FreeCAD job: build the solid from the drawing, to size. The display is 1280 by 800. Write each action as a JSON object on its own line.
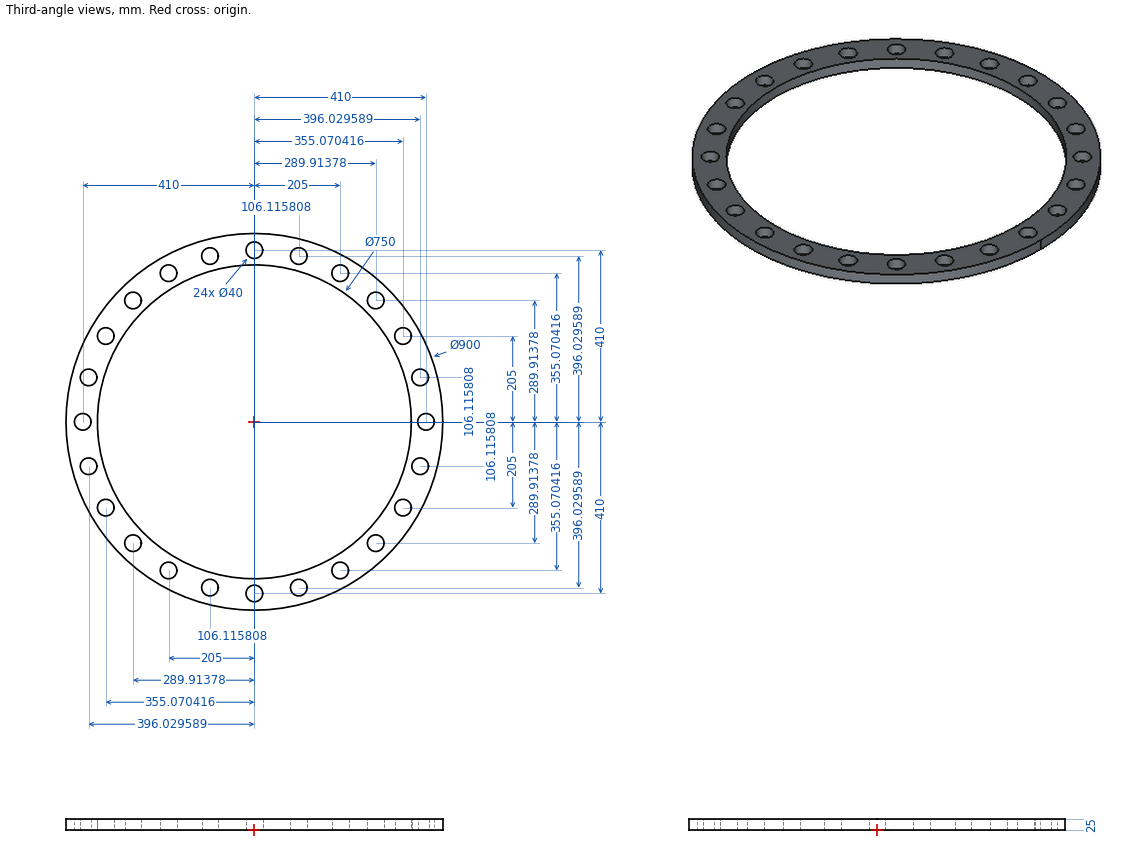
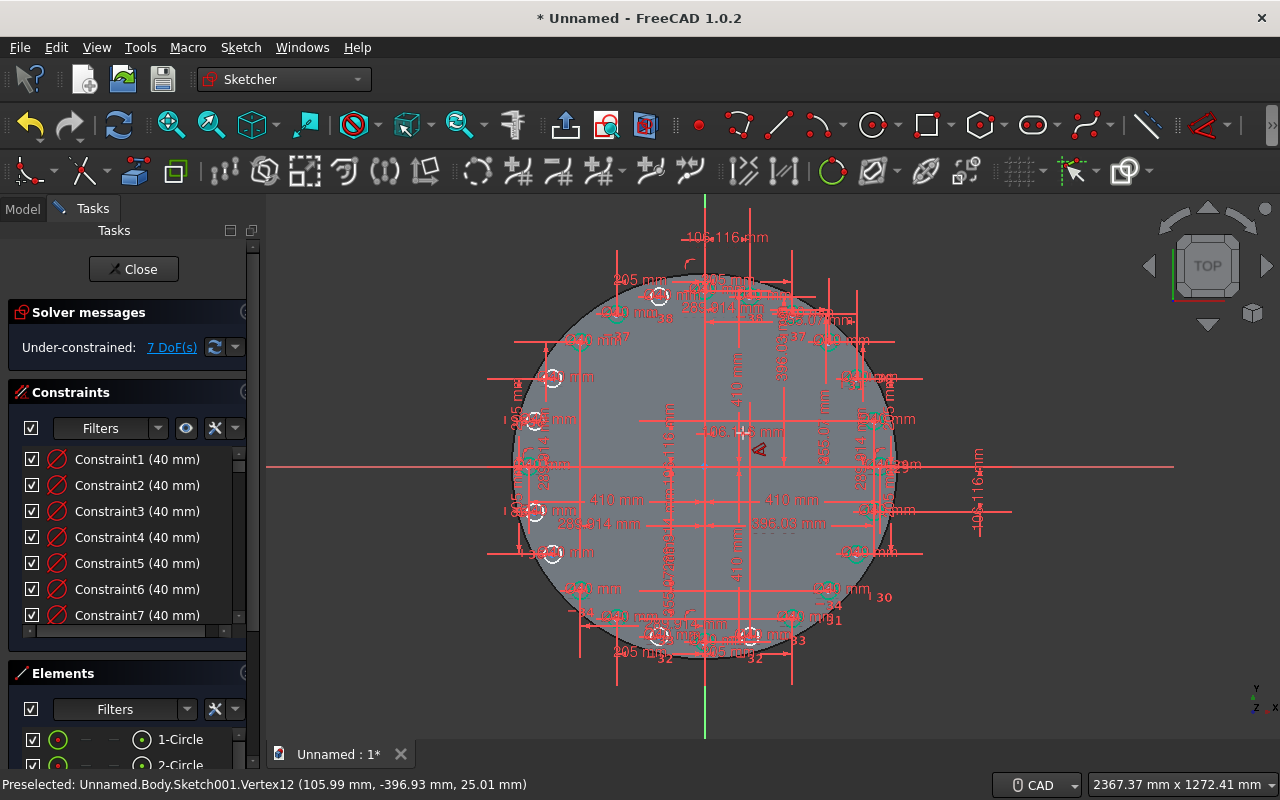
{"action": "left_click", "coordinate": [750, 637]}
{"action": "left_click", "coordinate": [784, 591]}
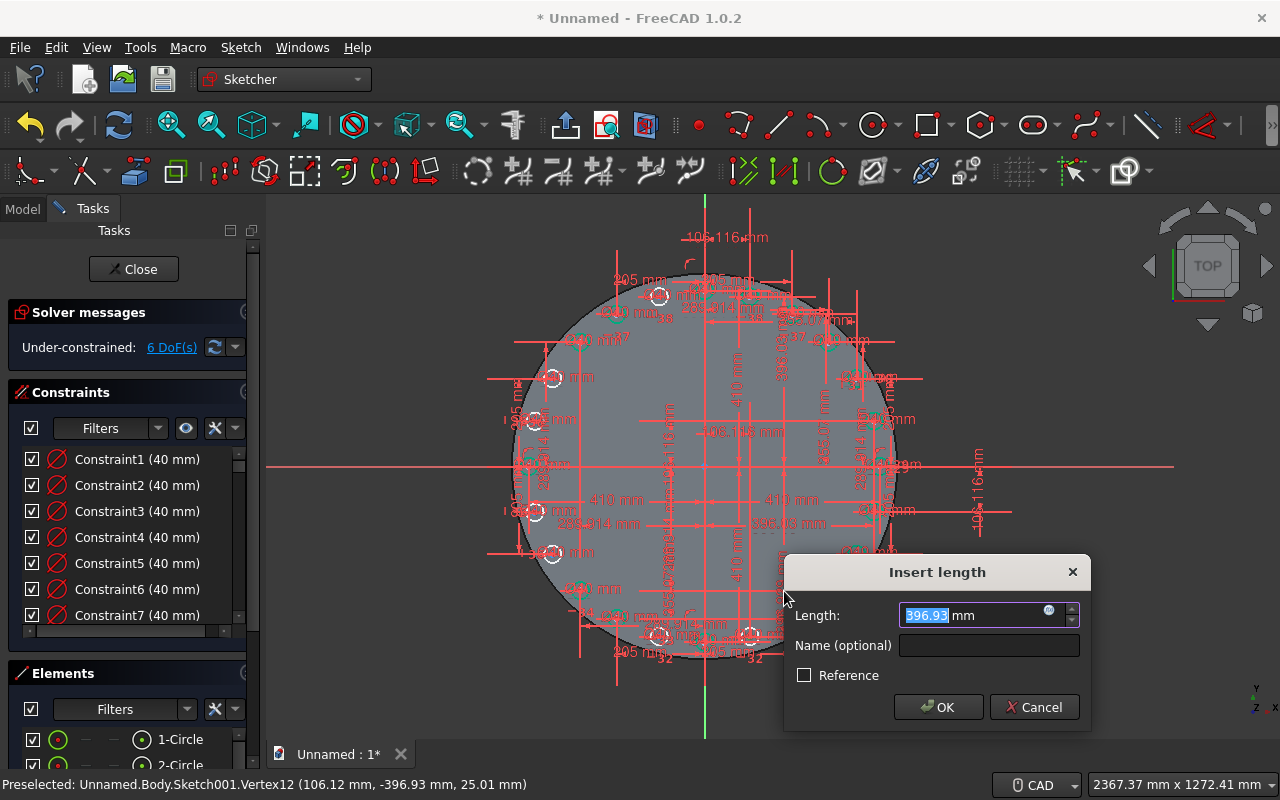
{"action": "type", "text": "396.029589"}
{"action": "key", "text": "Return"}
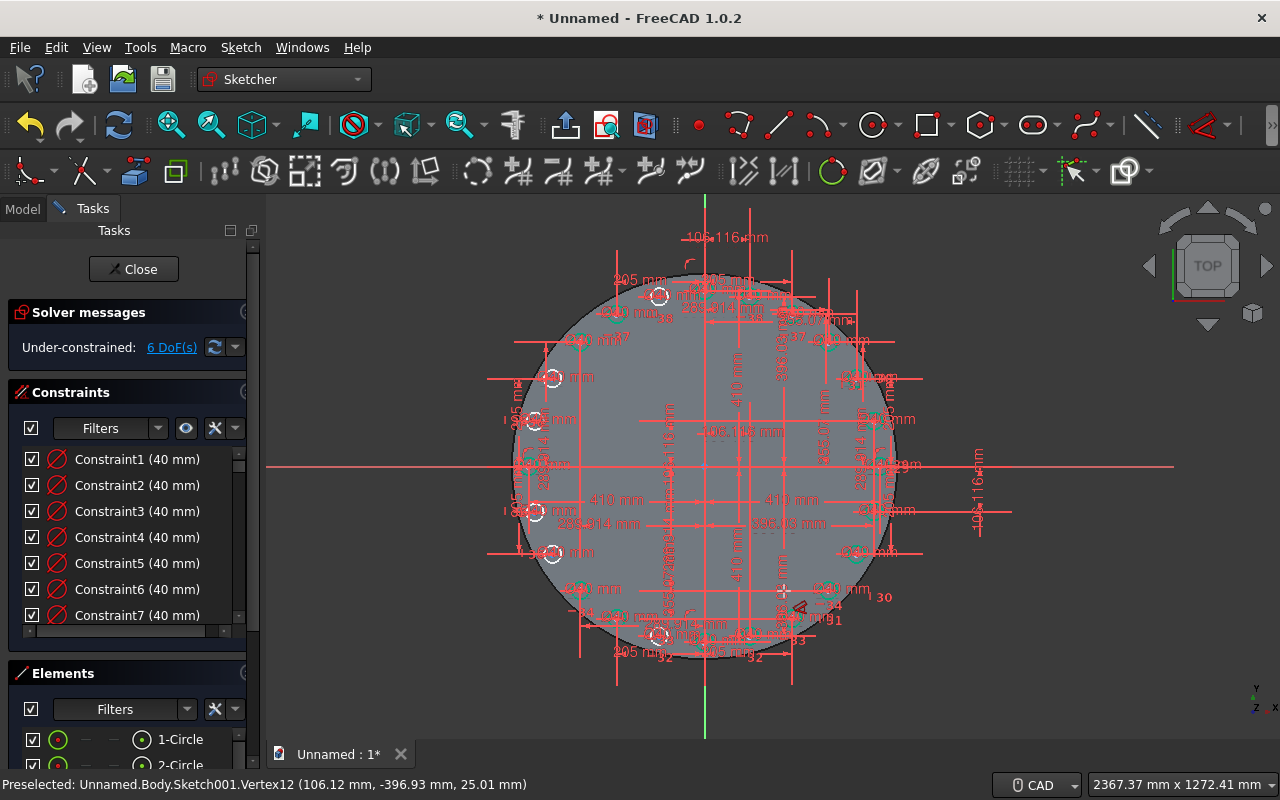
{"action": "left_click", "coordinate": [659, 636]}
{"action": "left_click", "coordinate": [682, 694]}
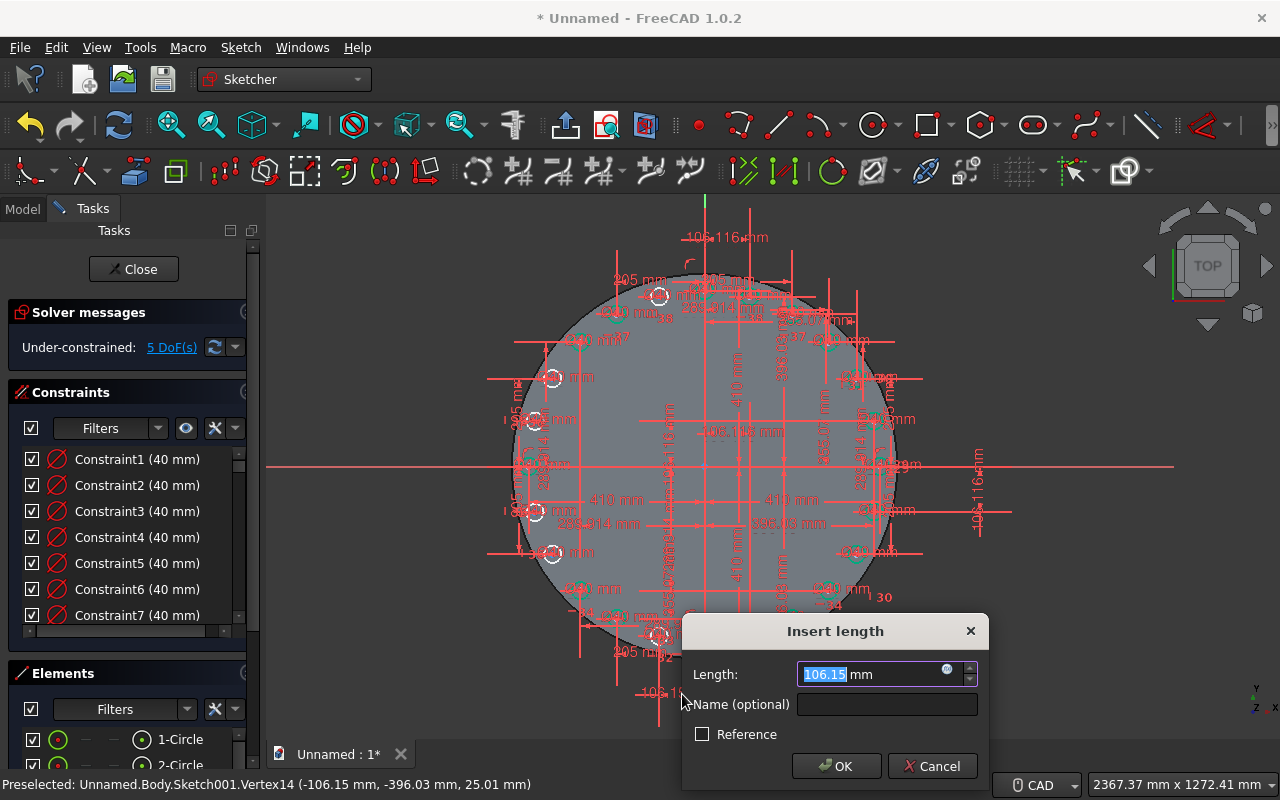
{"action": "type", "text": "106.115808"}
{"action": "key", "text": "Return"}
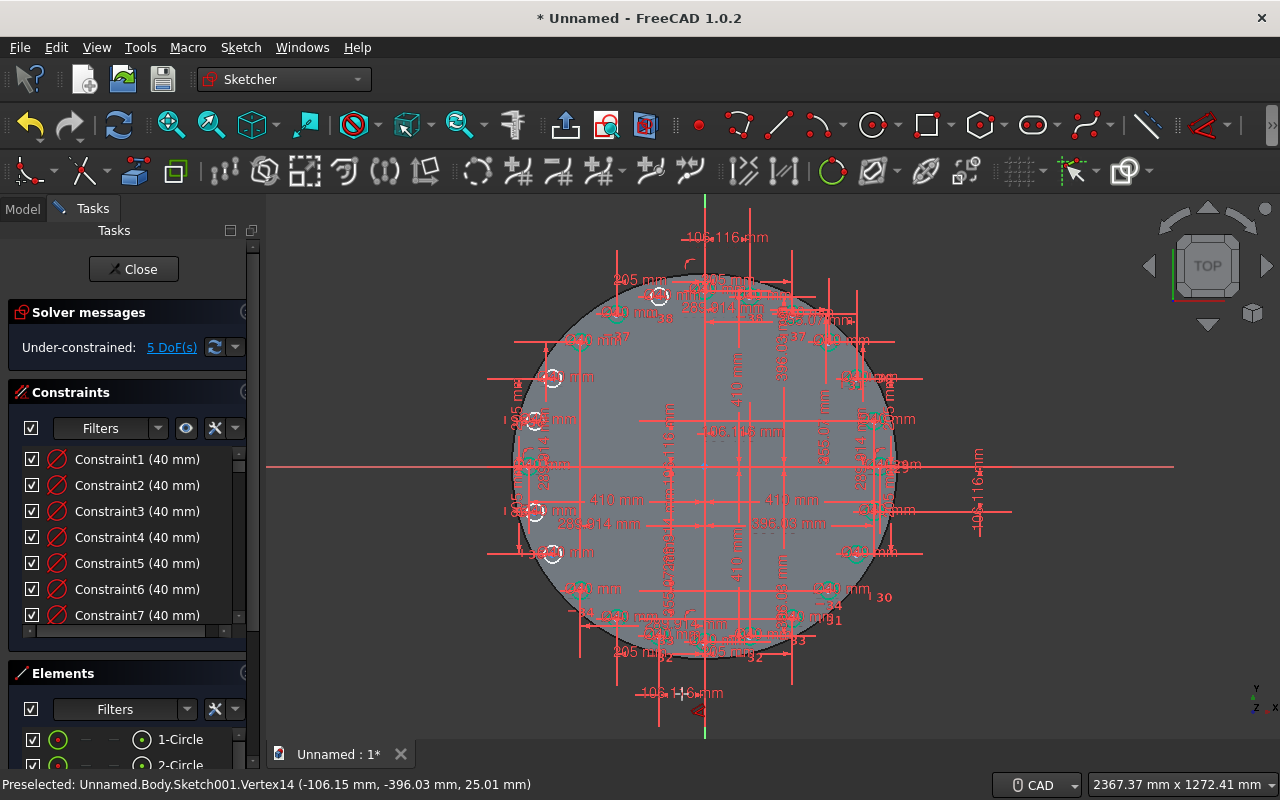
{"action": "left_click", "coordinate": [553, 554]}
{"action": "left_click", "coordinate": [594, 612]}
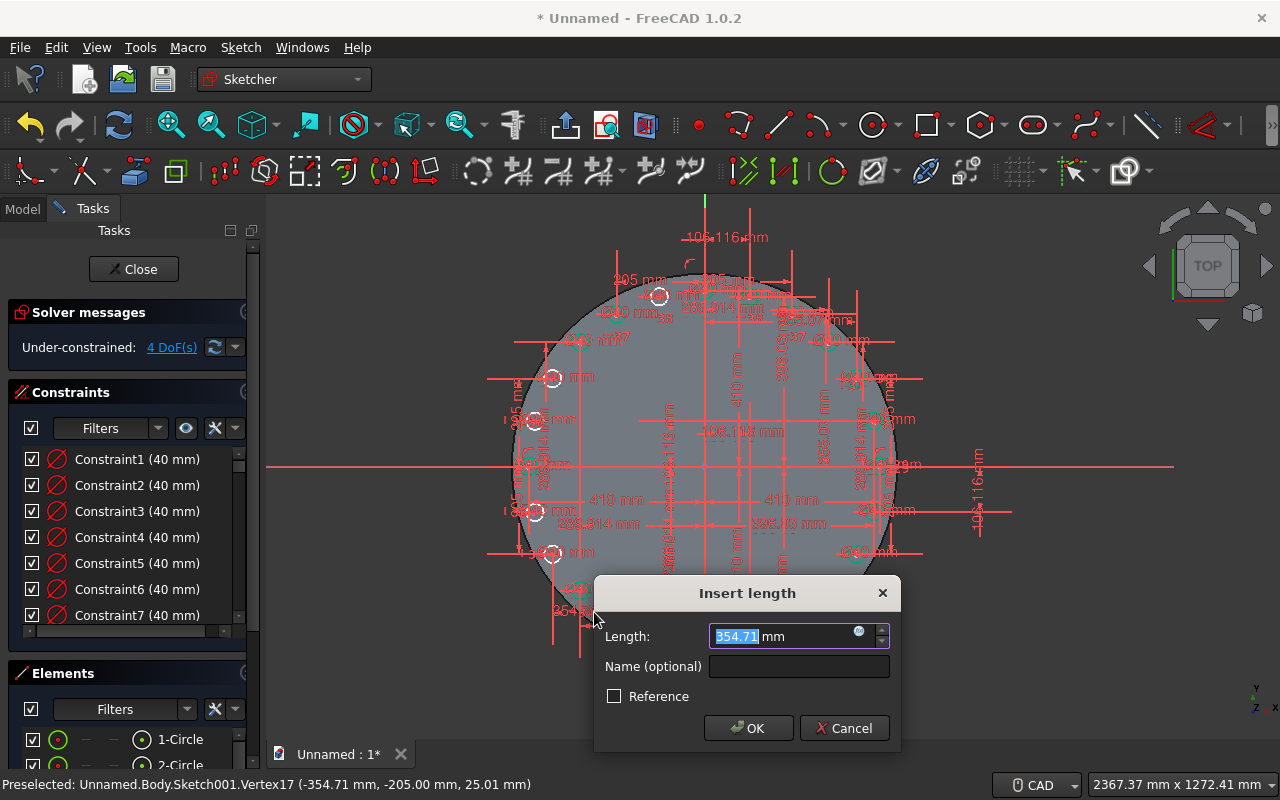
{"action": "type", "text": "355.070416"}
{"action": "key", "text": "Return"}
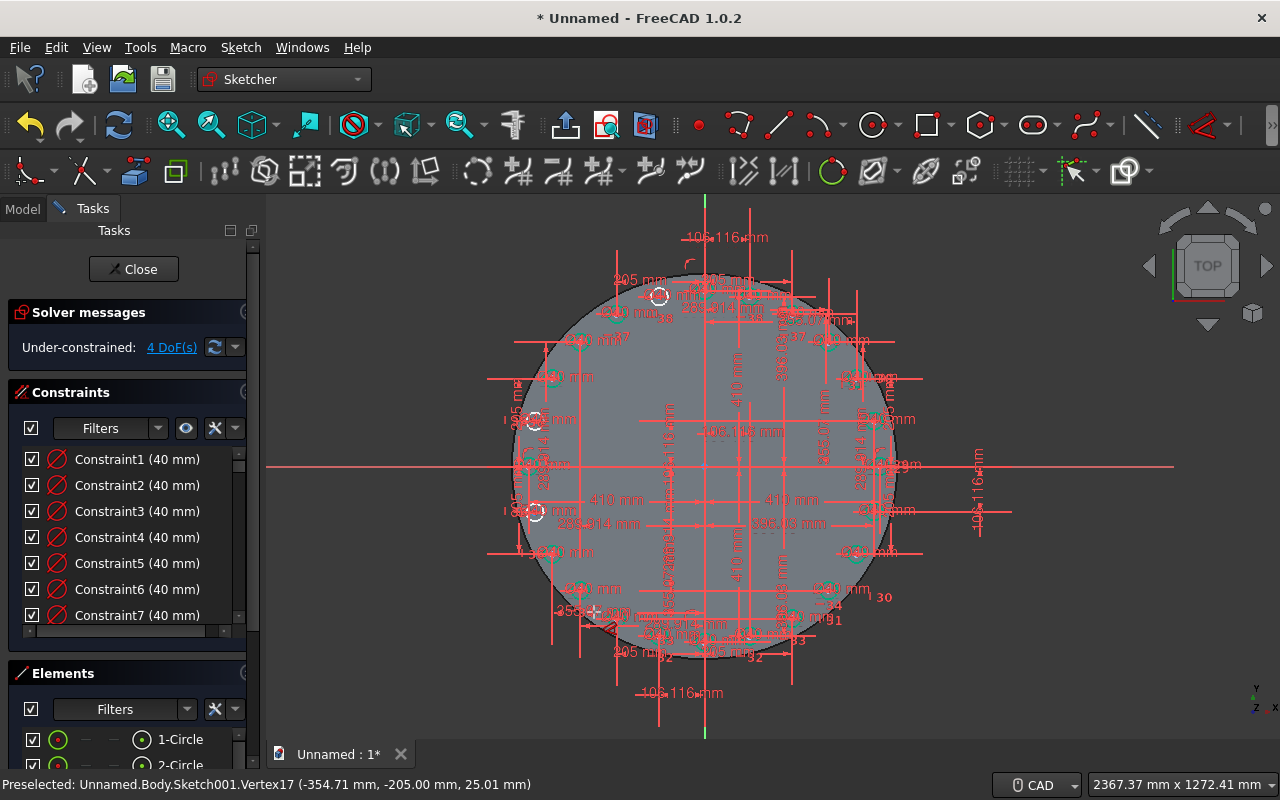
{"action": "left_click", "coordinate": [535, 512]}
{"action": "left_click", "coordinate": [581, 546]}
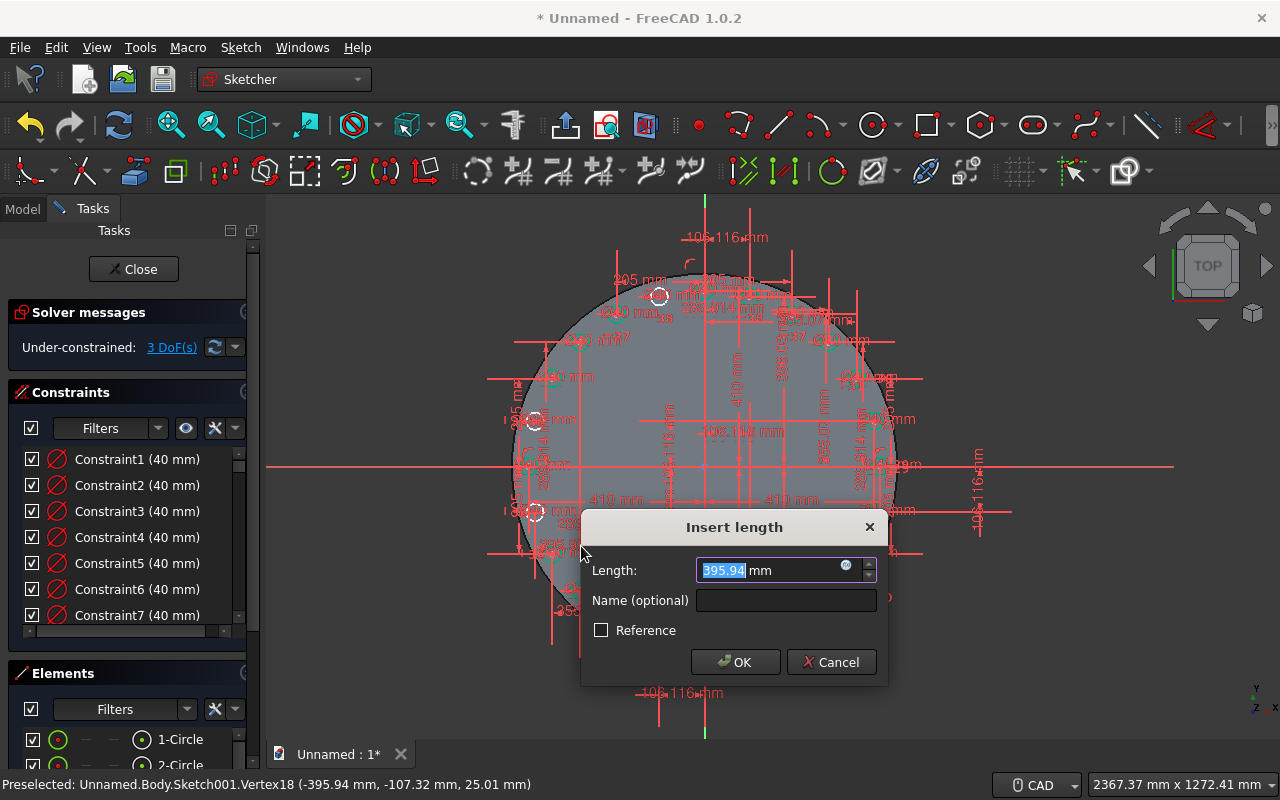
{"action": "type", "text": "396.029589"}
{"action": "key", "text": "Return"}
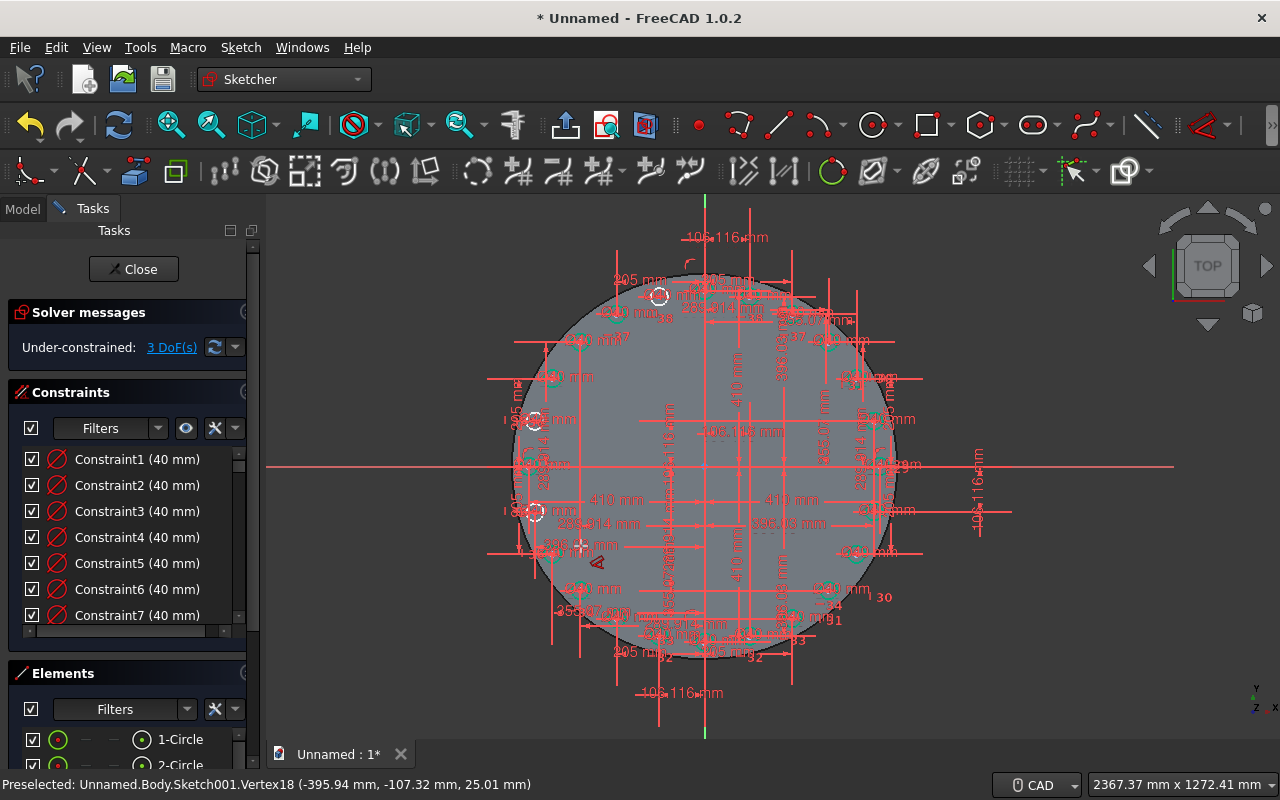
{"action": "left_click", "coordinate": [535, 512]}
{"action": "left_click", "coordinate": [429, 489]}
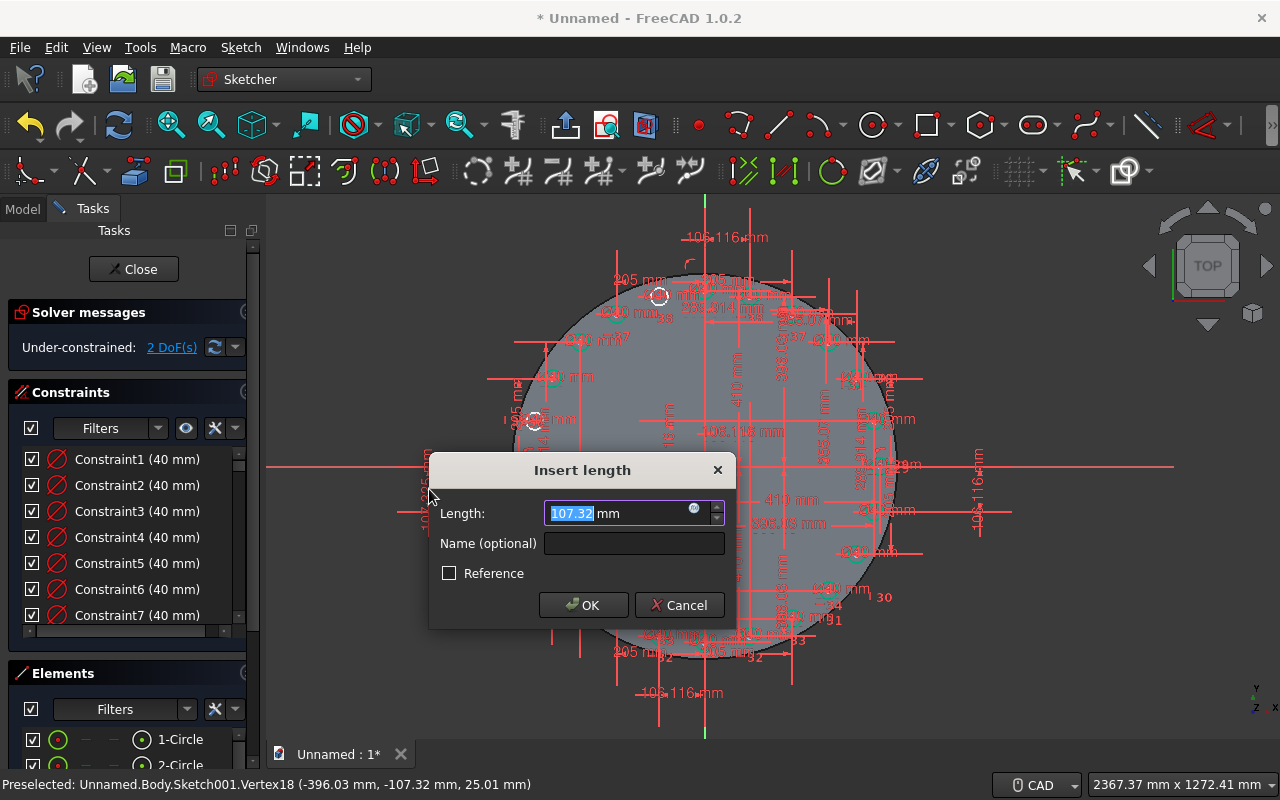
{"action": "type", "text": "106.115808"}
{"action": "key", "text": "Return"}